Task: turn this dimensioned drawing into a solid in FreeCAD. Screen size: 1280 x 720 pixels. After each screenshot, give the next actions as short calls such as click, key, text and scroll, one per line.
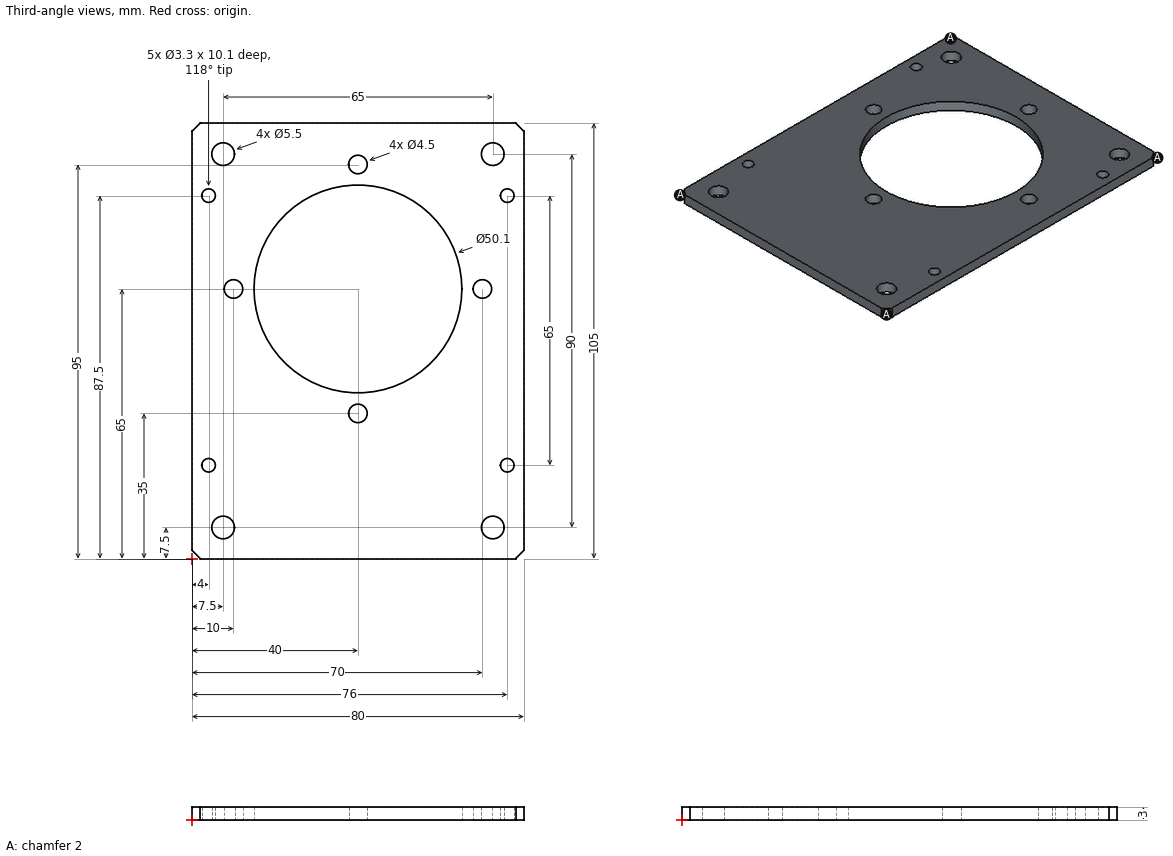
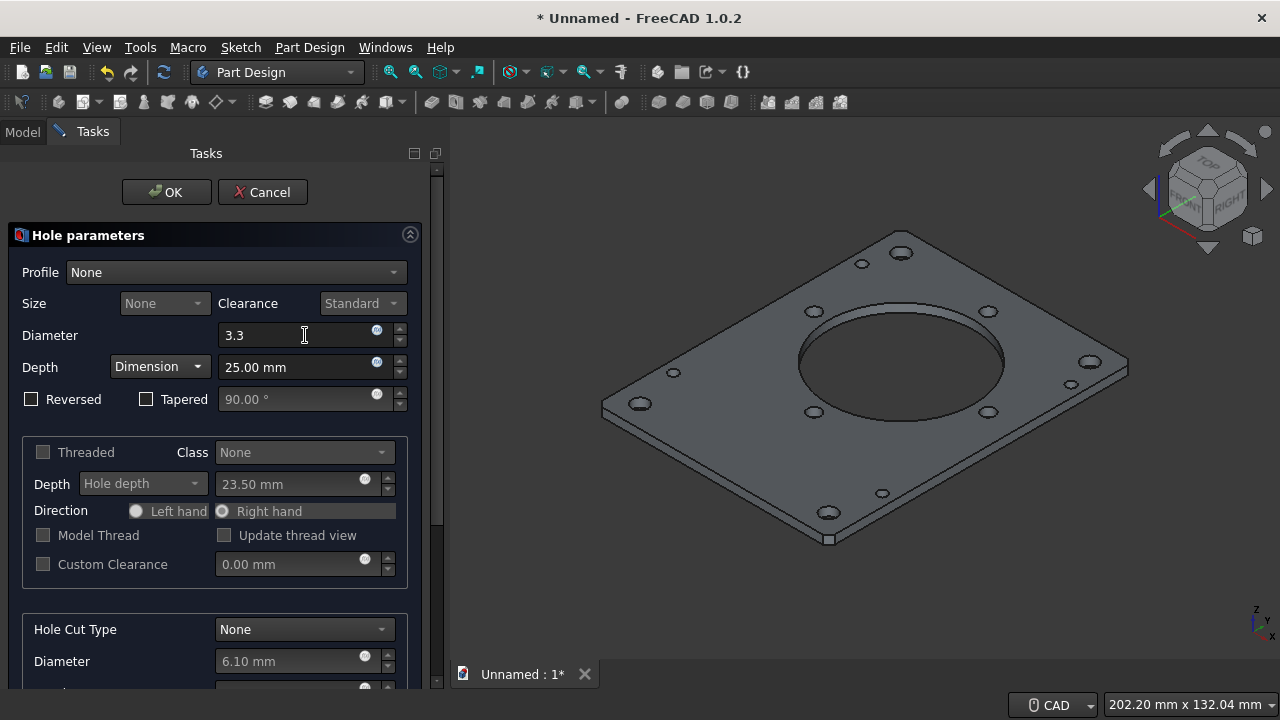
triple_click(305, 367)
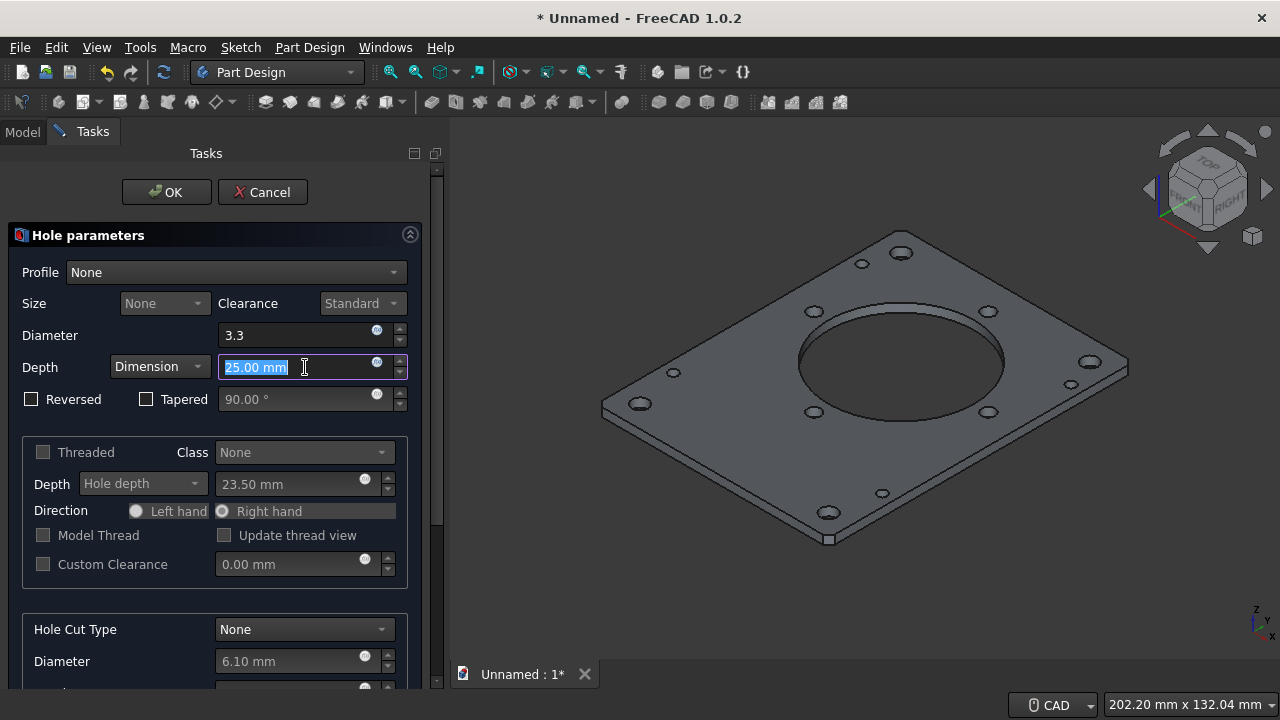
text(10.1)
key(Tab)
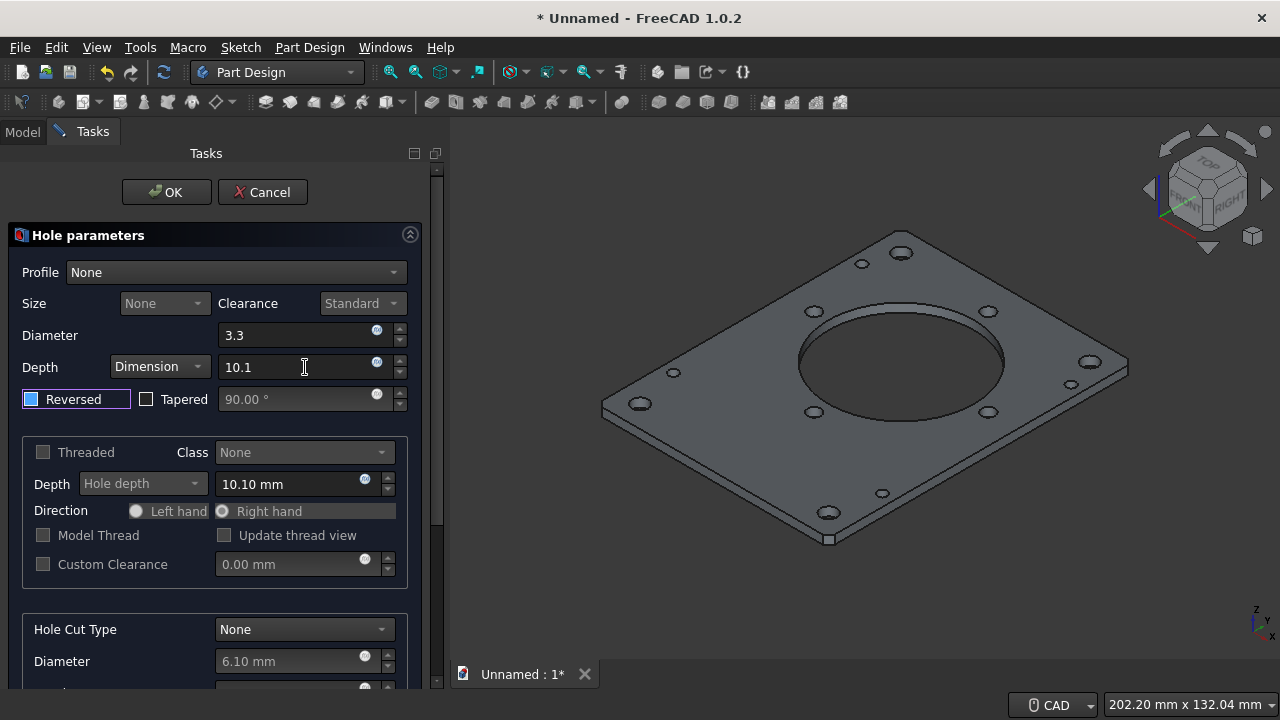
click(167, 192)